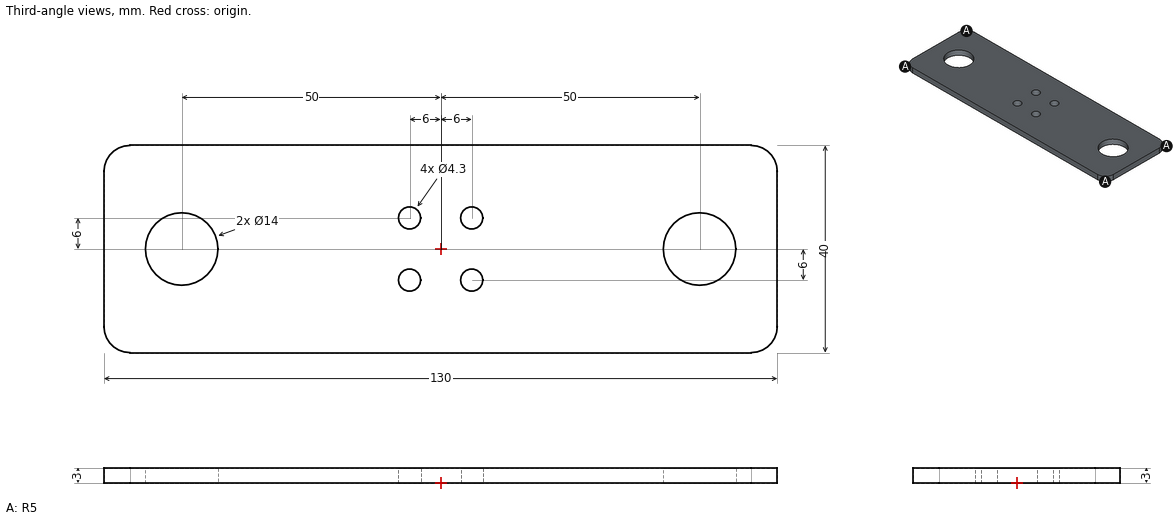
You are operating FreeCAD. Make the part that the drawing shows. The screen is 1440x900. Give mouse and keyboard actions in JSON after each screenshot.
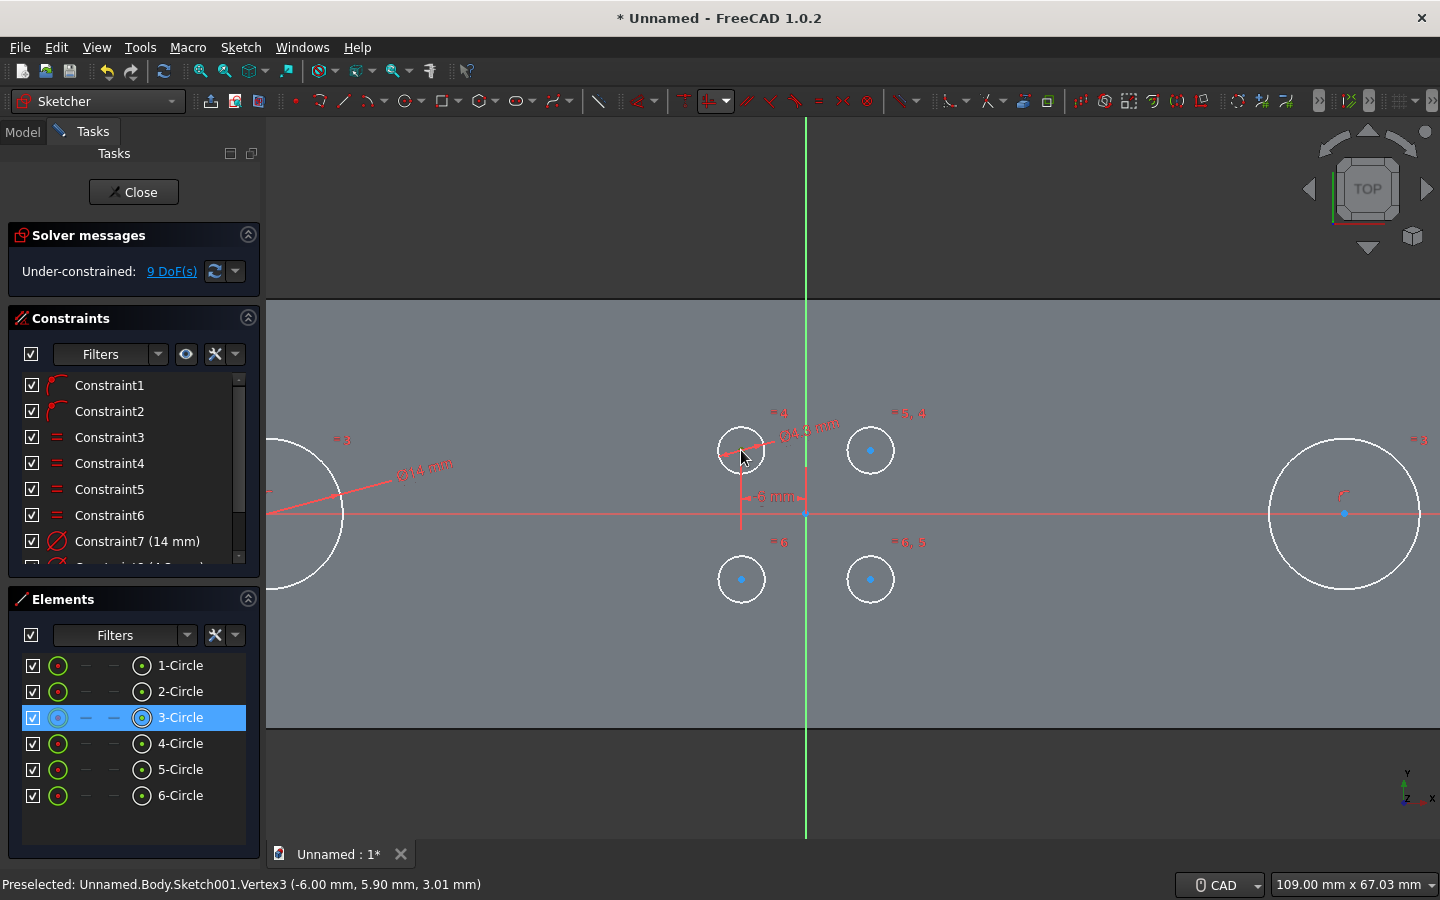
{"action": "key", "text": "i"}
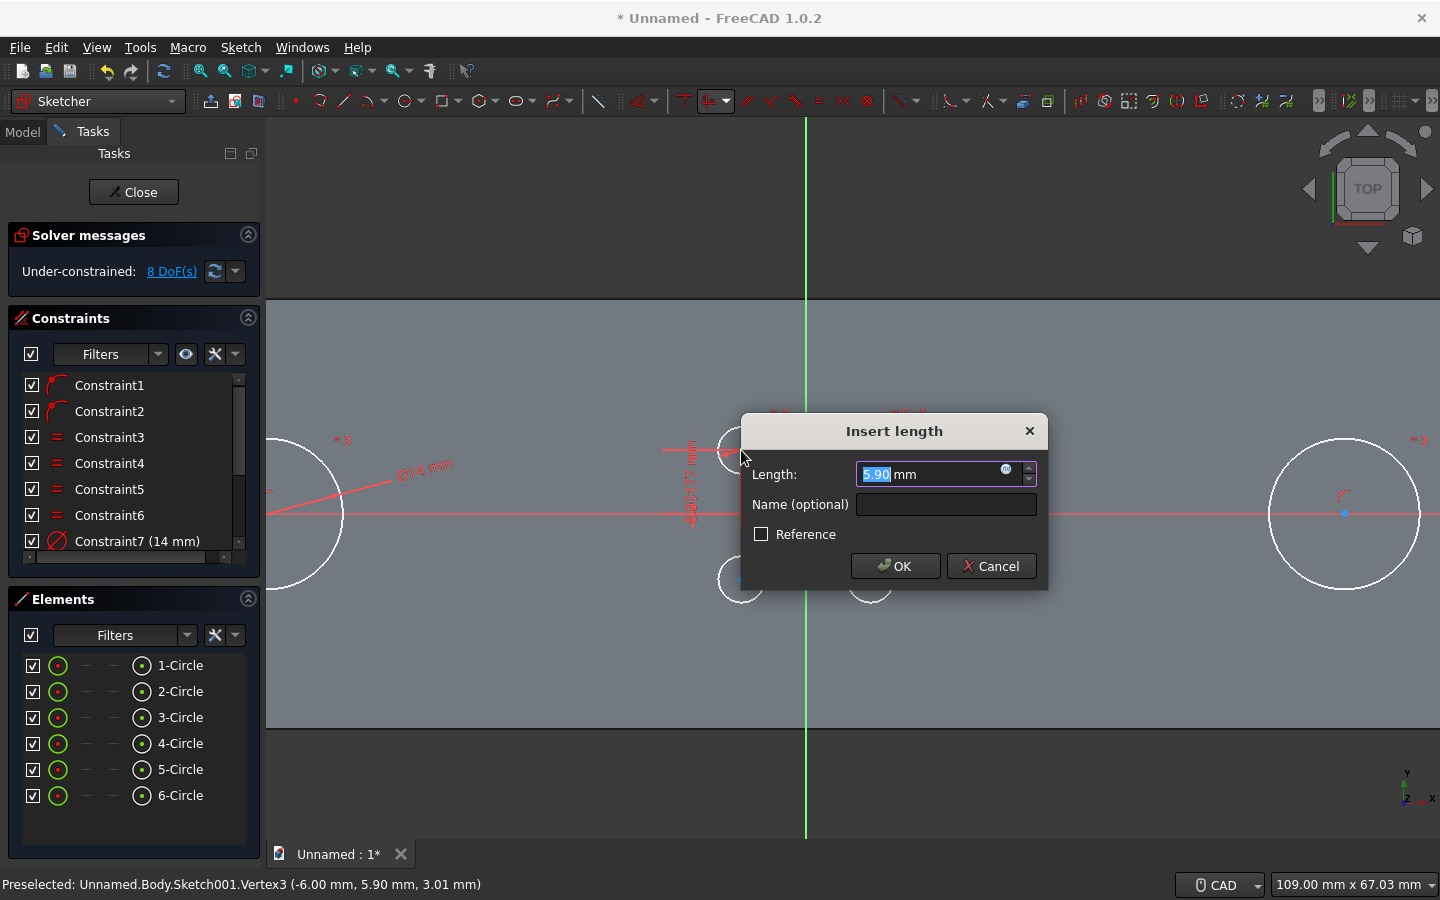
{"action": "type", "text": "6"}
{"action": "key", "text": "Return"}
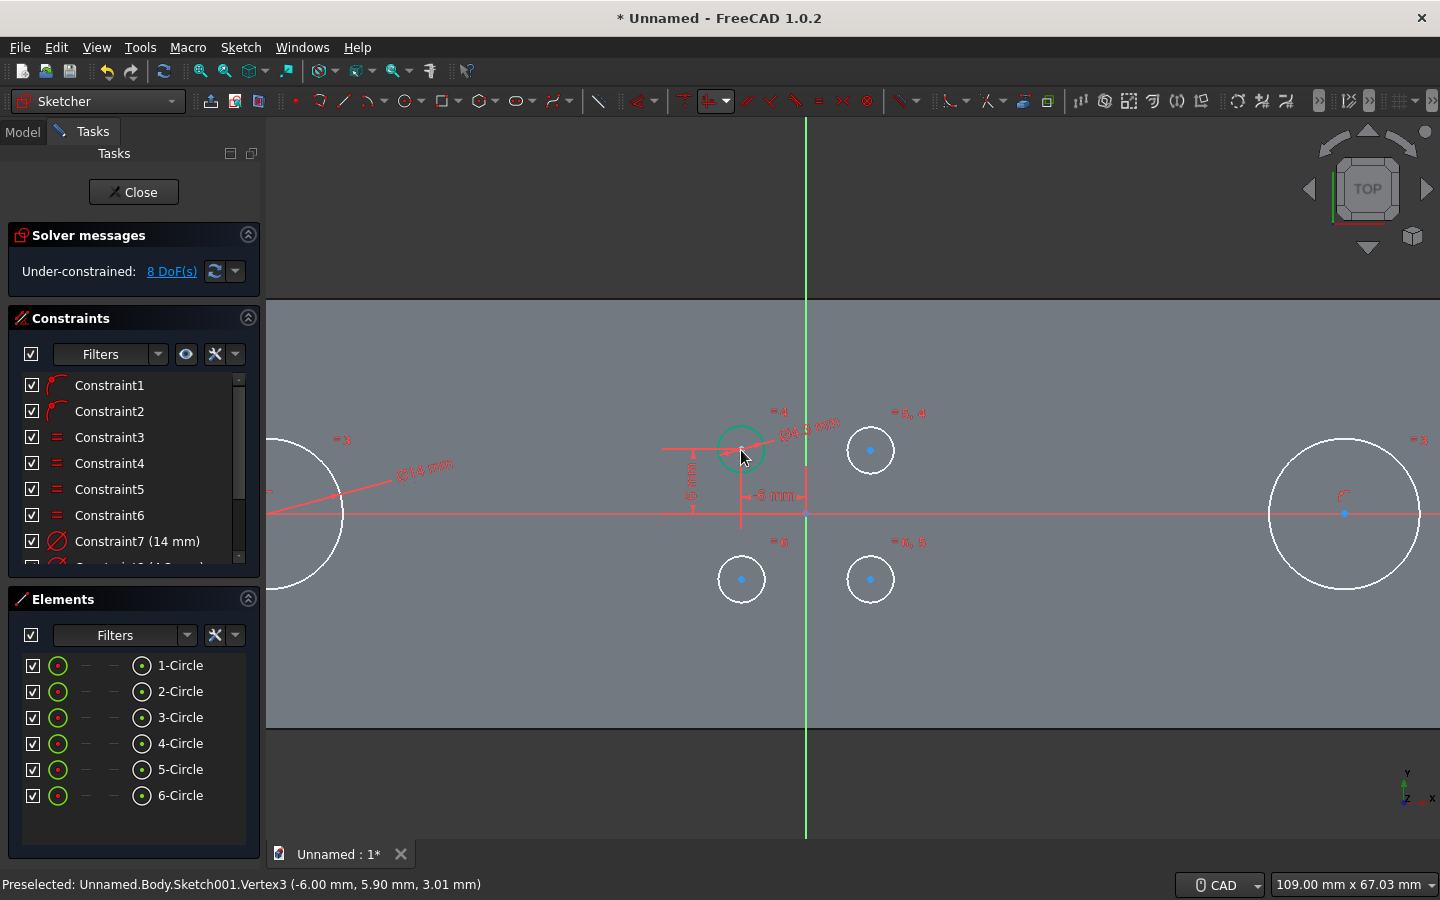
{"action": "left_click", "coordinate": [871, 450]}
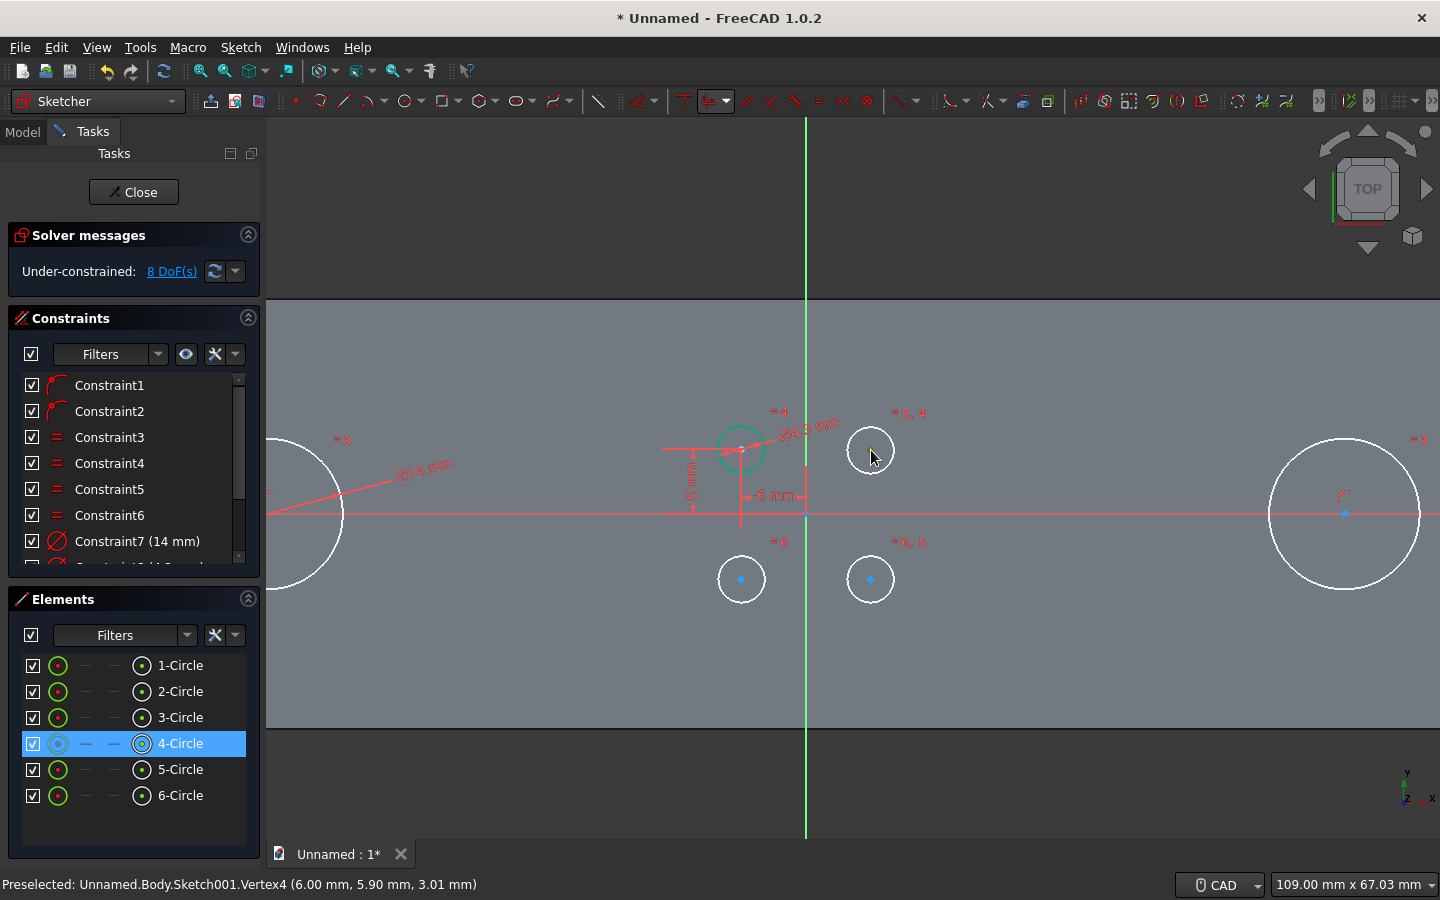
{"action": "key", "text": "l"}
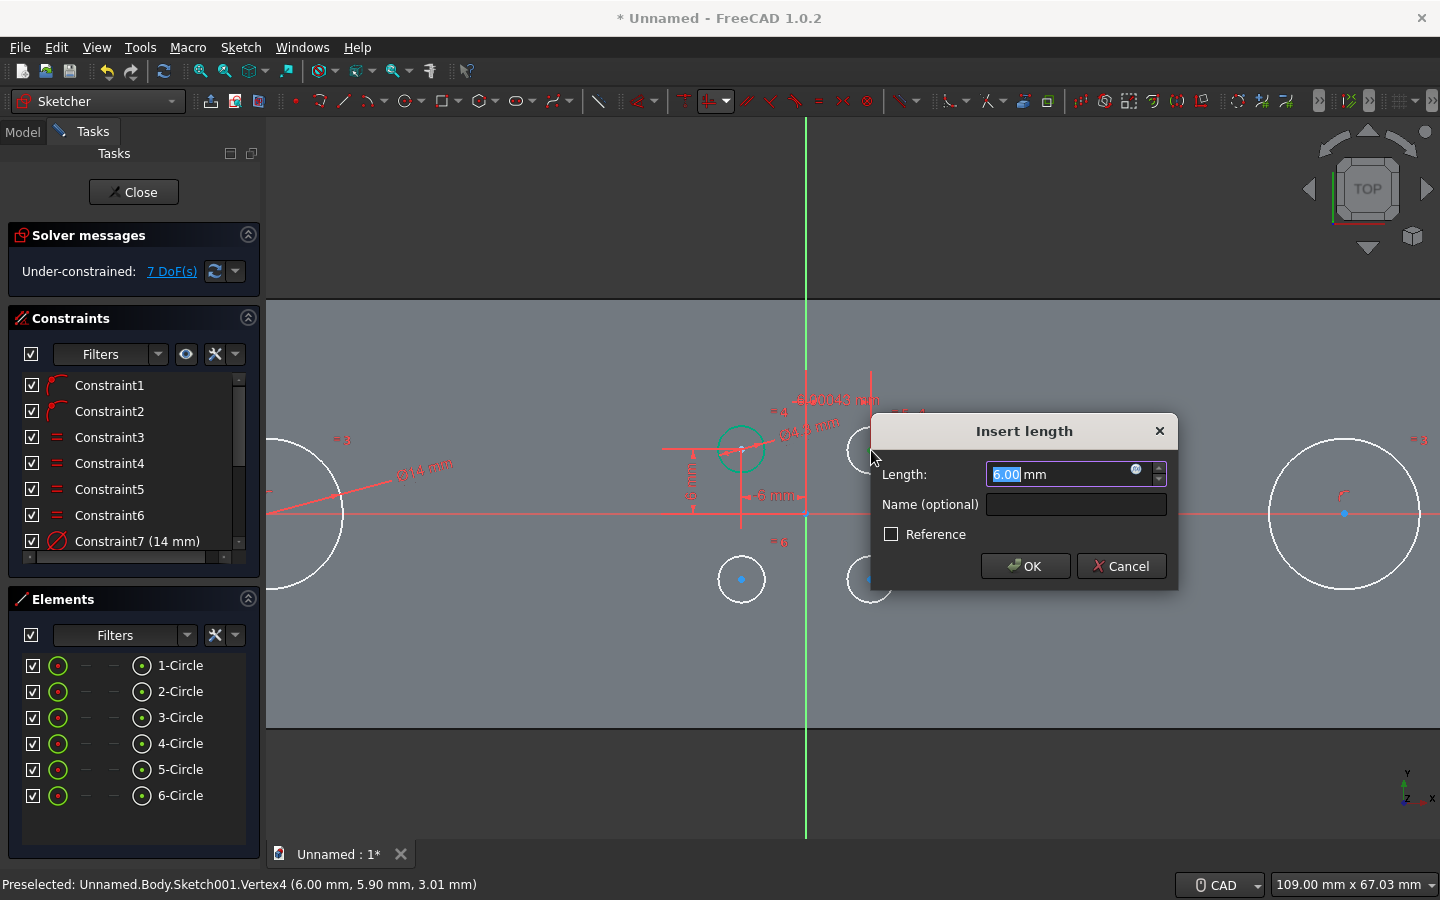
{"action": "type", "text": "6"}
{"action": "key", "text": "Return"}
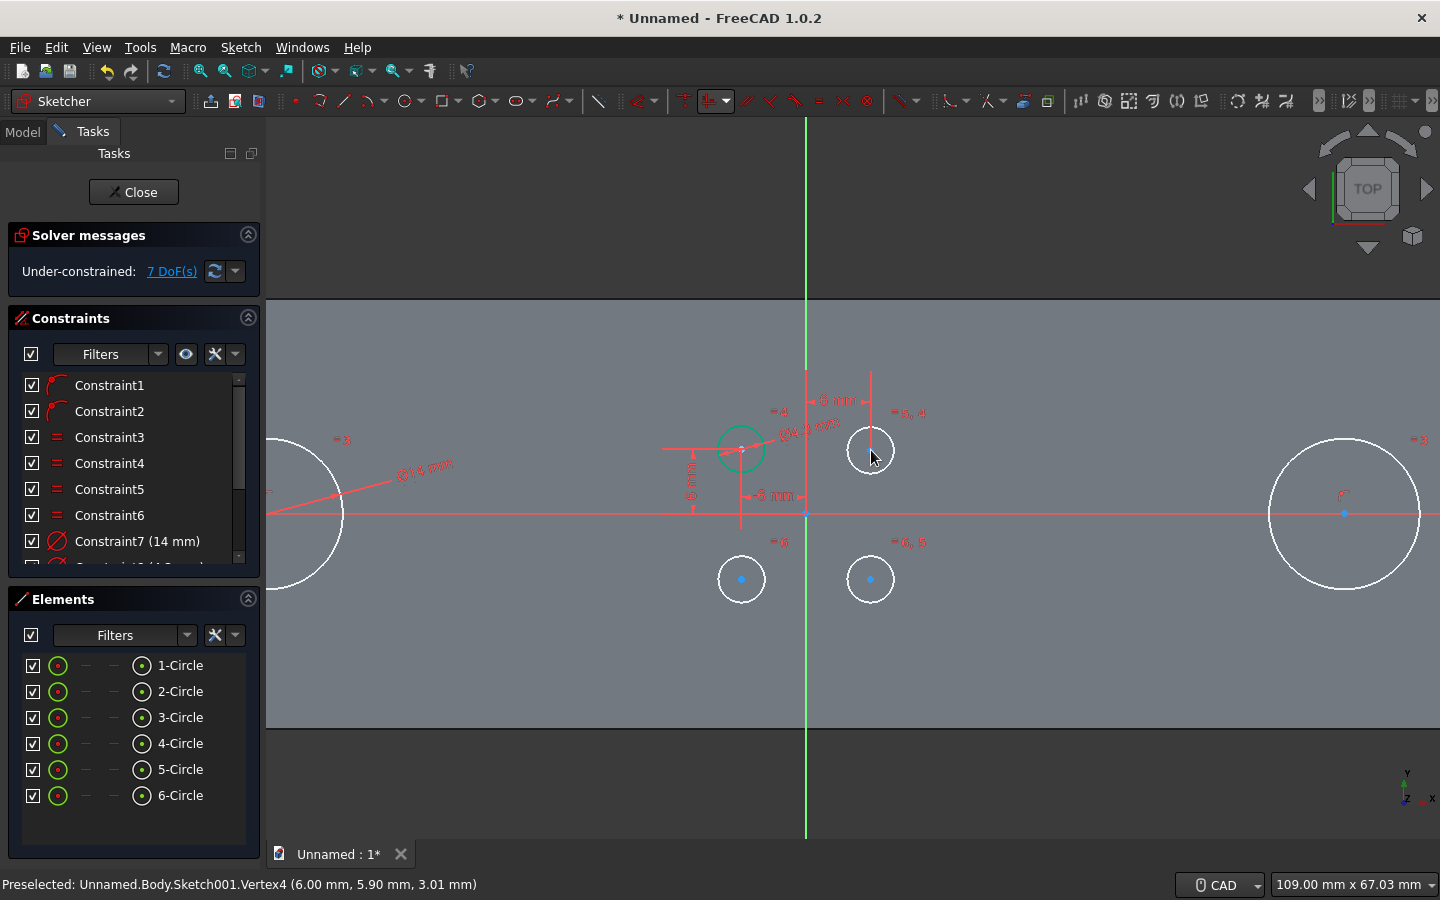
{"action": "left_click", "coordinate": [871, 450]}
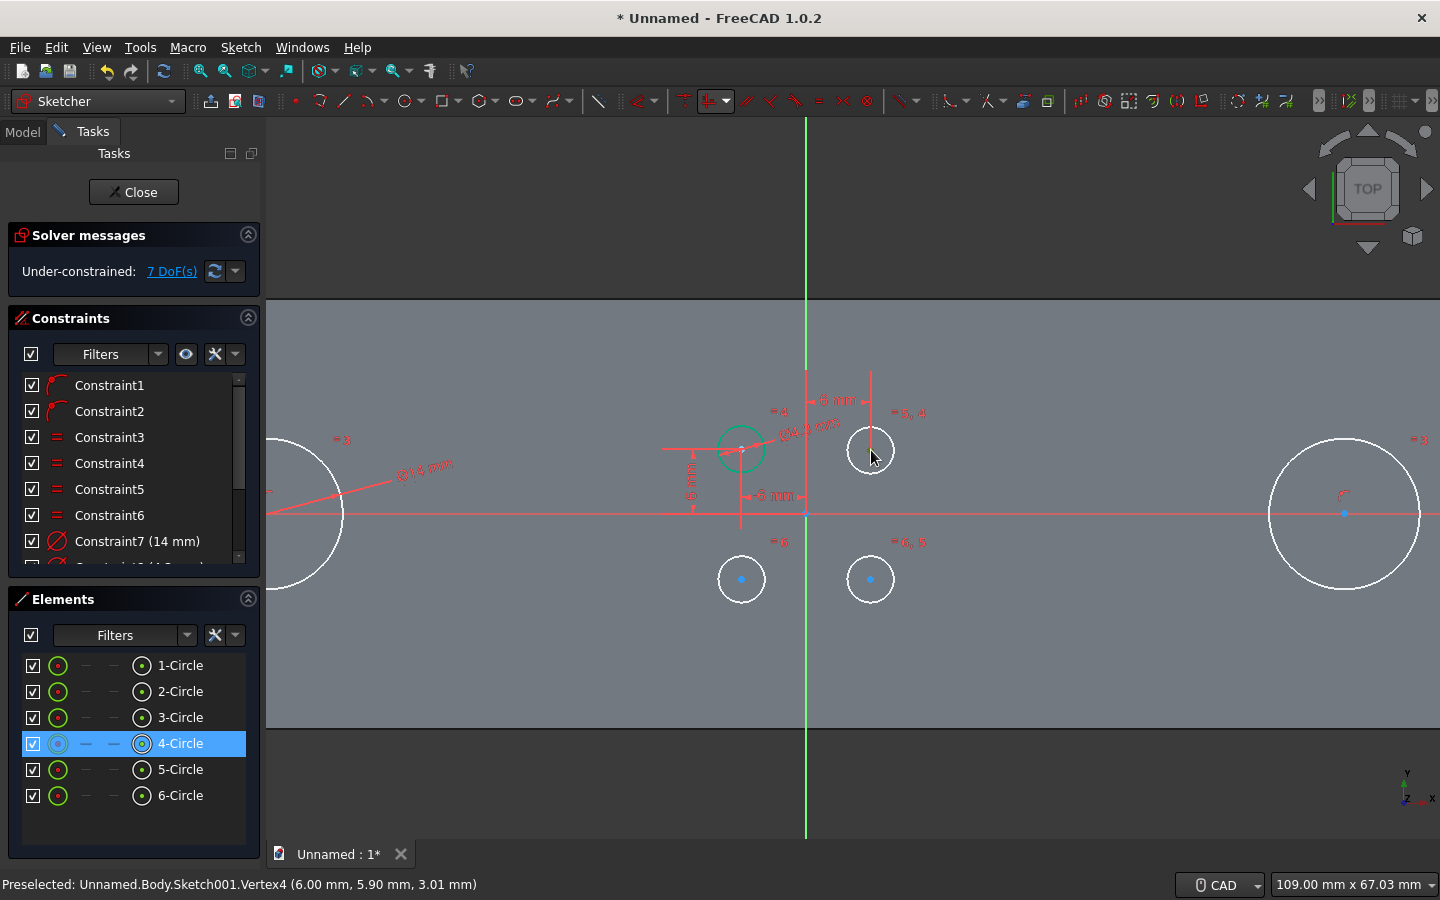
{"action": "key", "text": "i"}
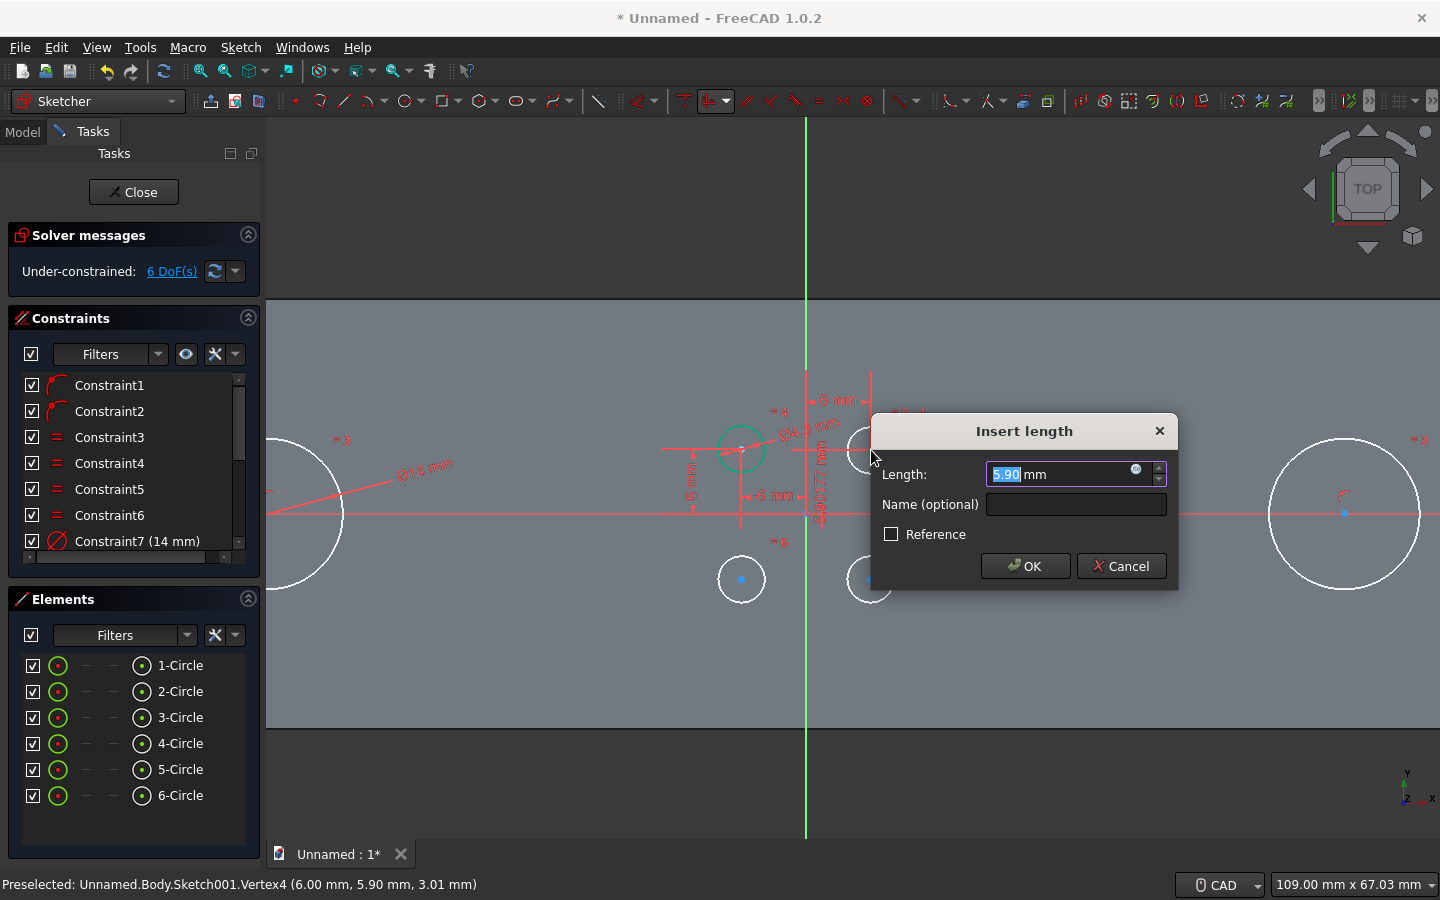
{"action": "type", "text": "6"}
{"action": "key", "text": "Return"}